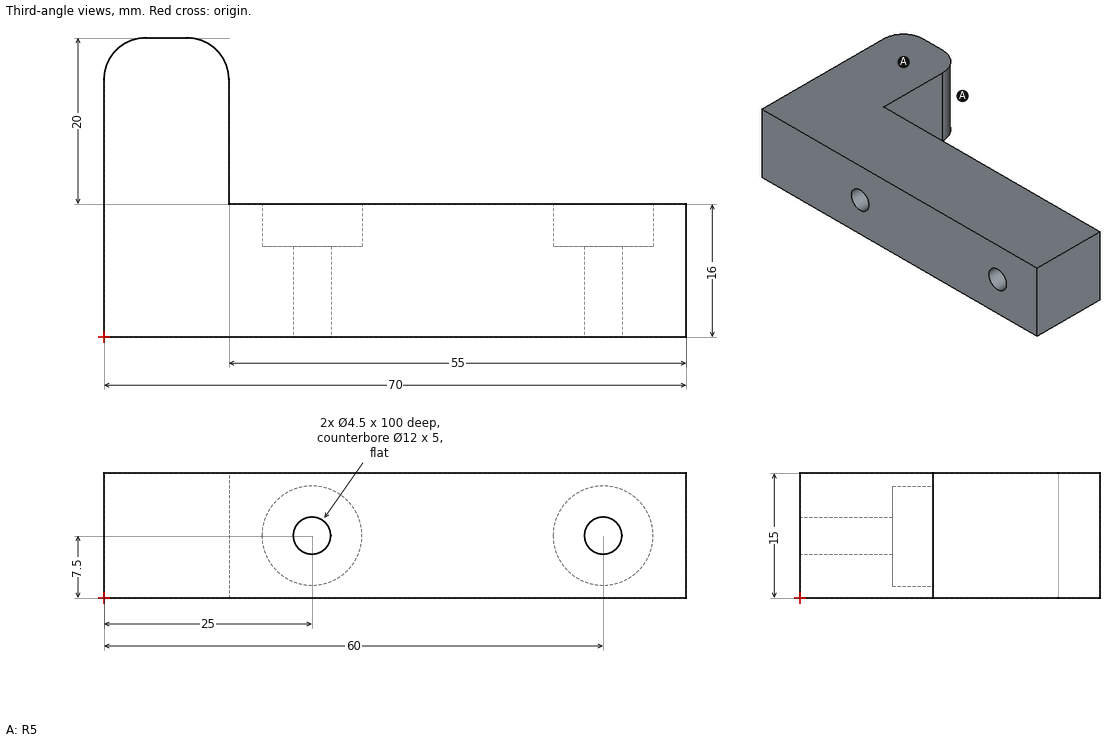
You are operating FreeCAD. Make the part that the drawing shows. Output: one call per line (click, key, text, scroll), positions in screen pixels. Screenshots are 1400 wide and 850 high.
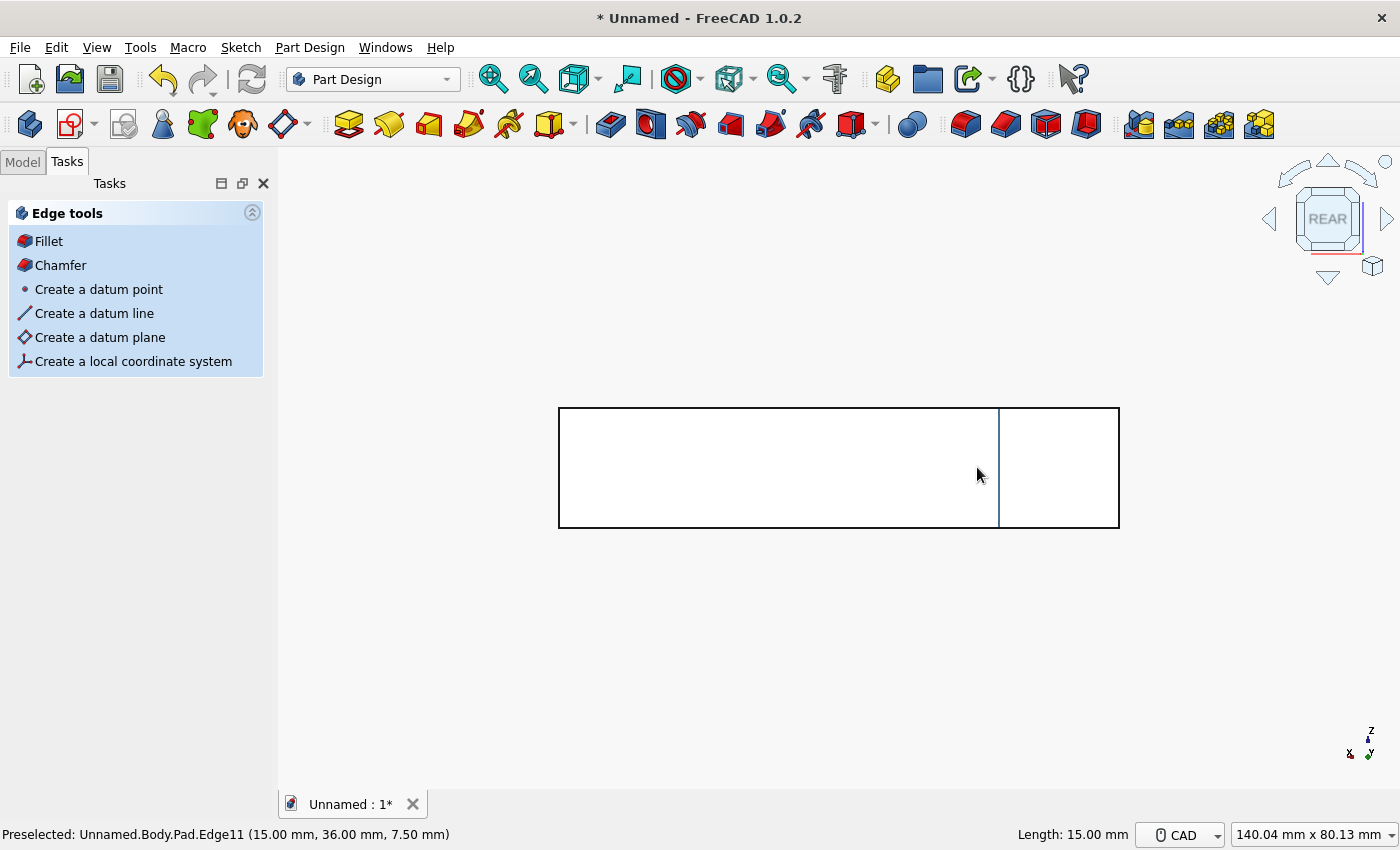
click(1119, 467, ctrl)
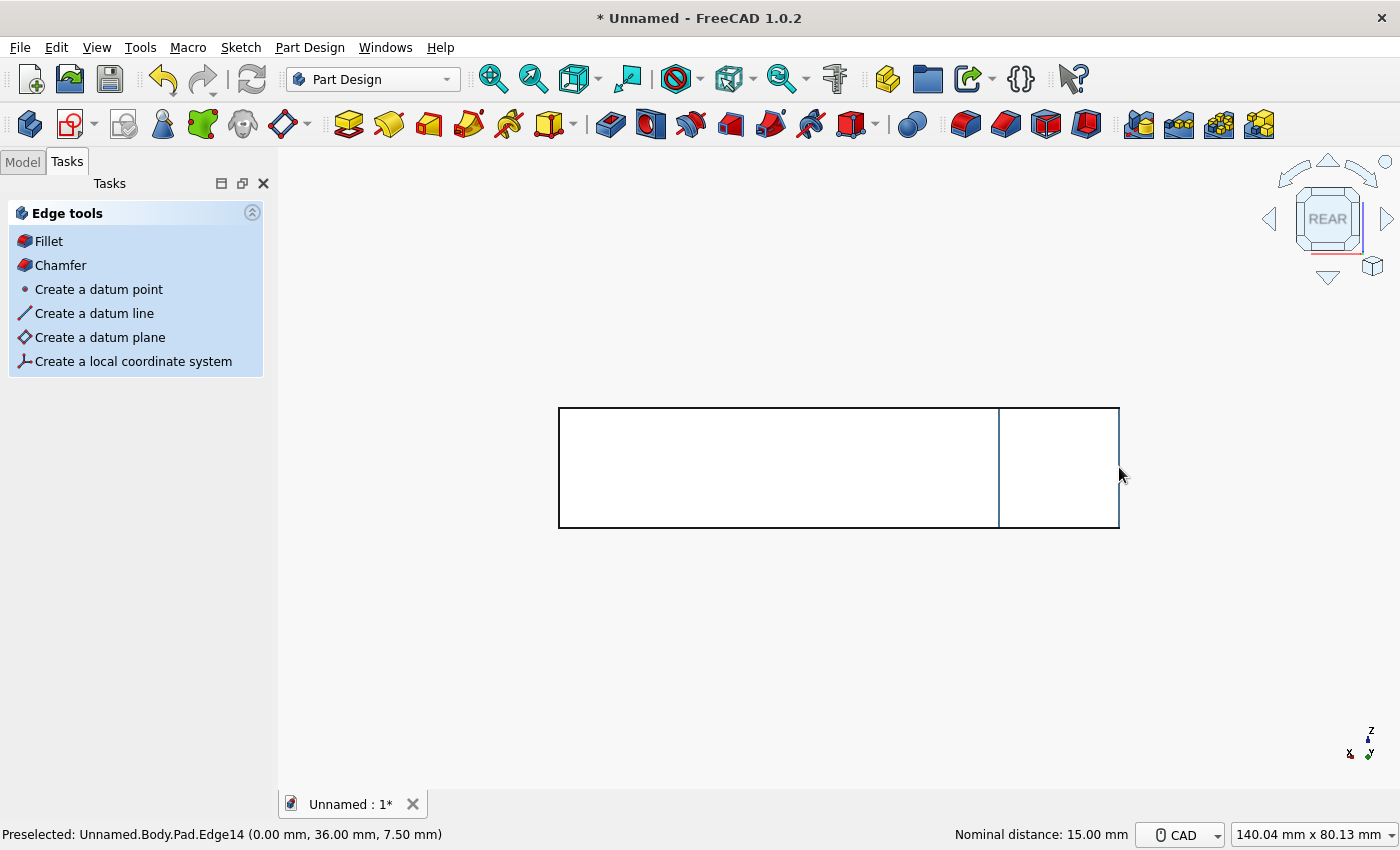
click(966, 124)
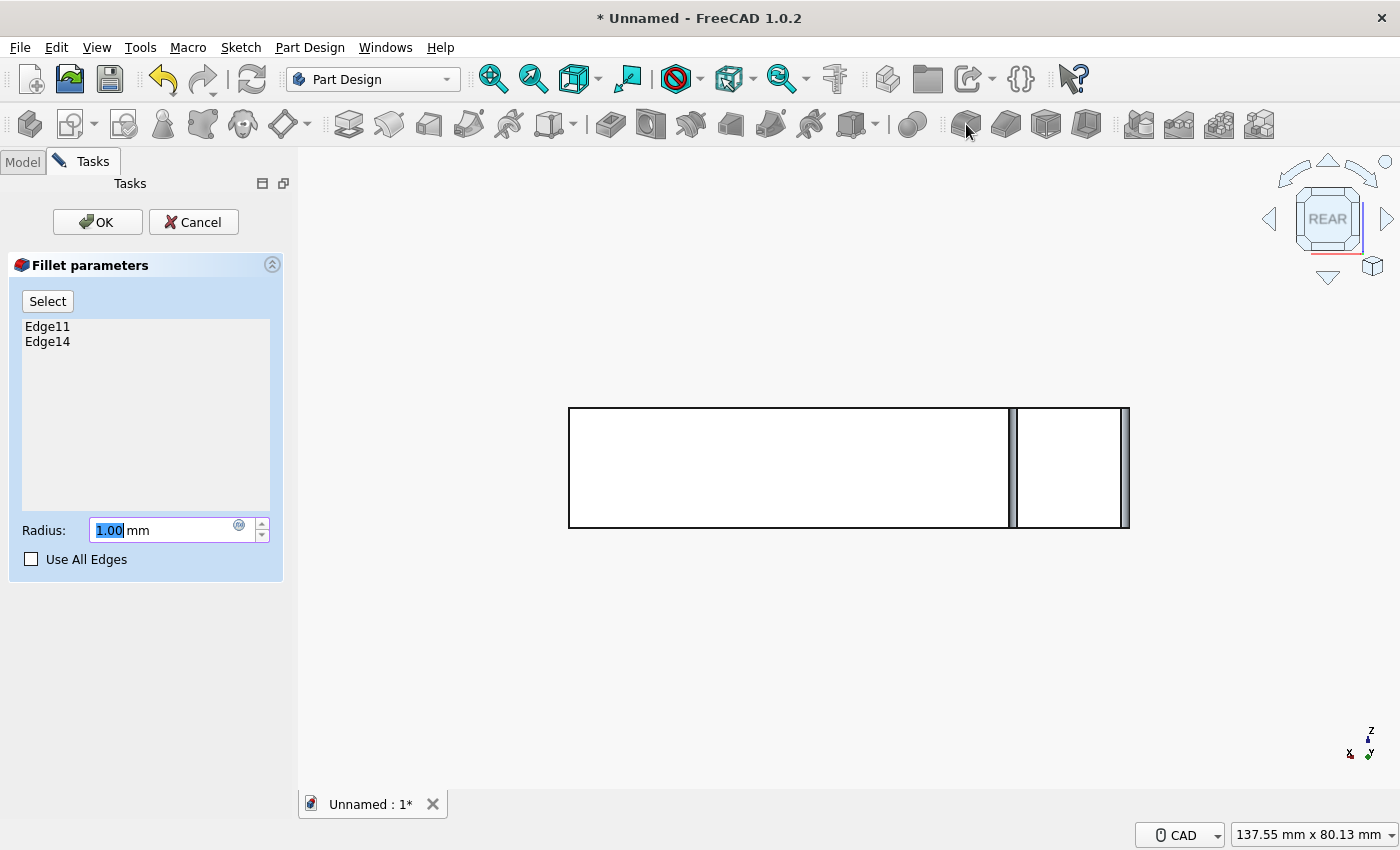
text(5)
key(Tab)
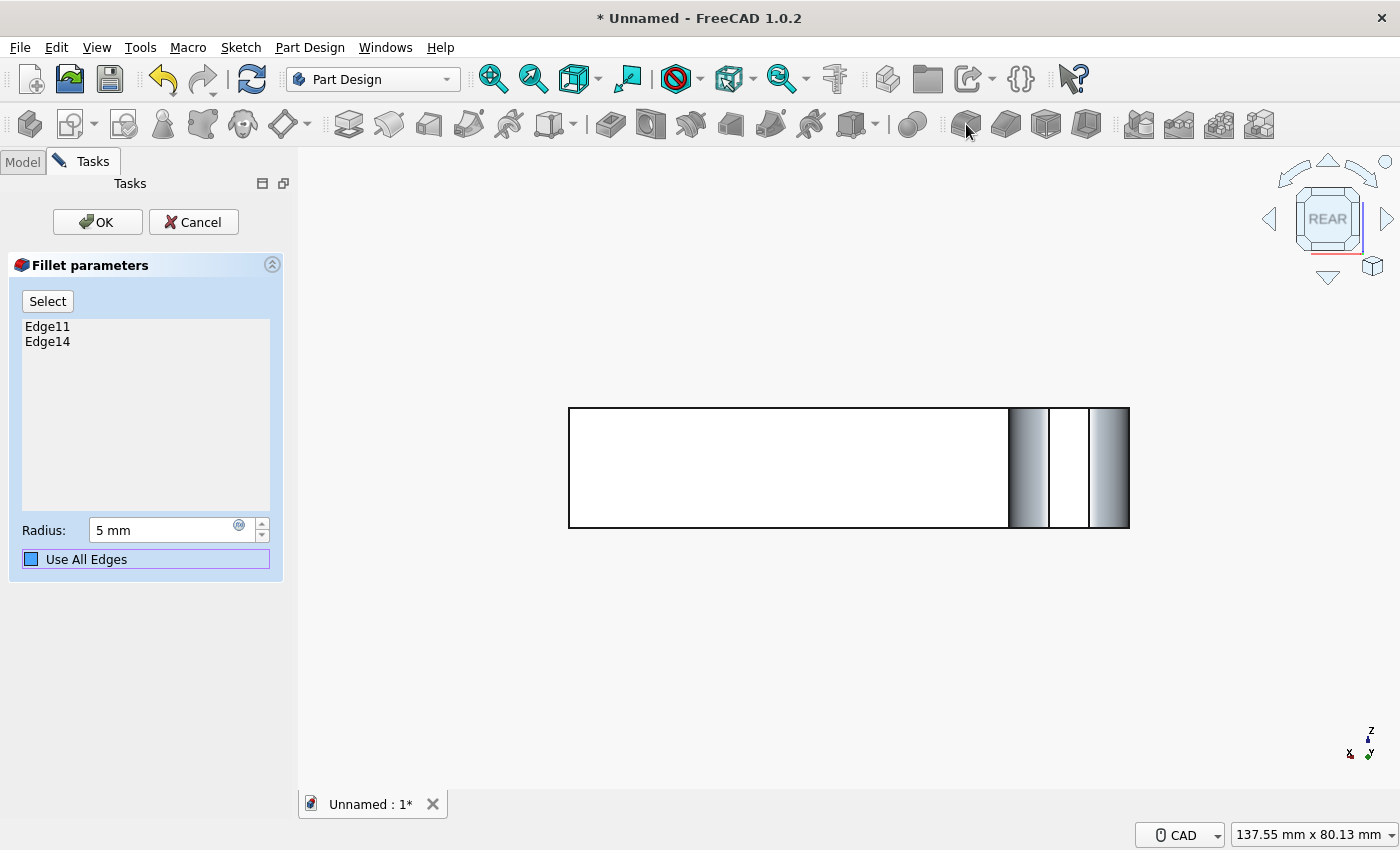
click(98, 222)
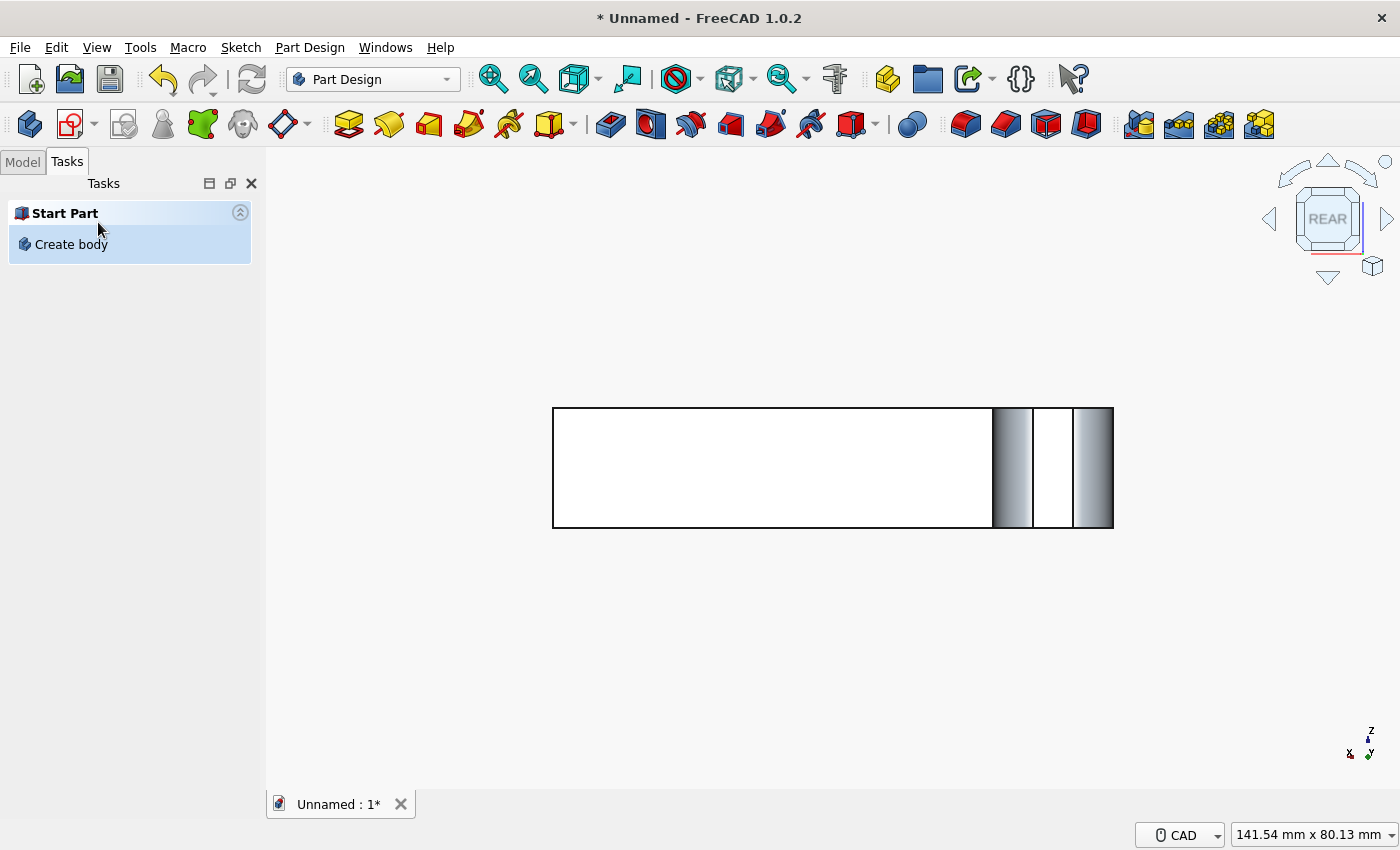
click(647, 467)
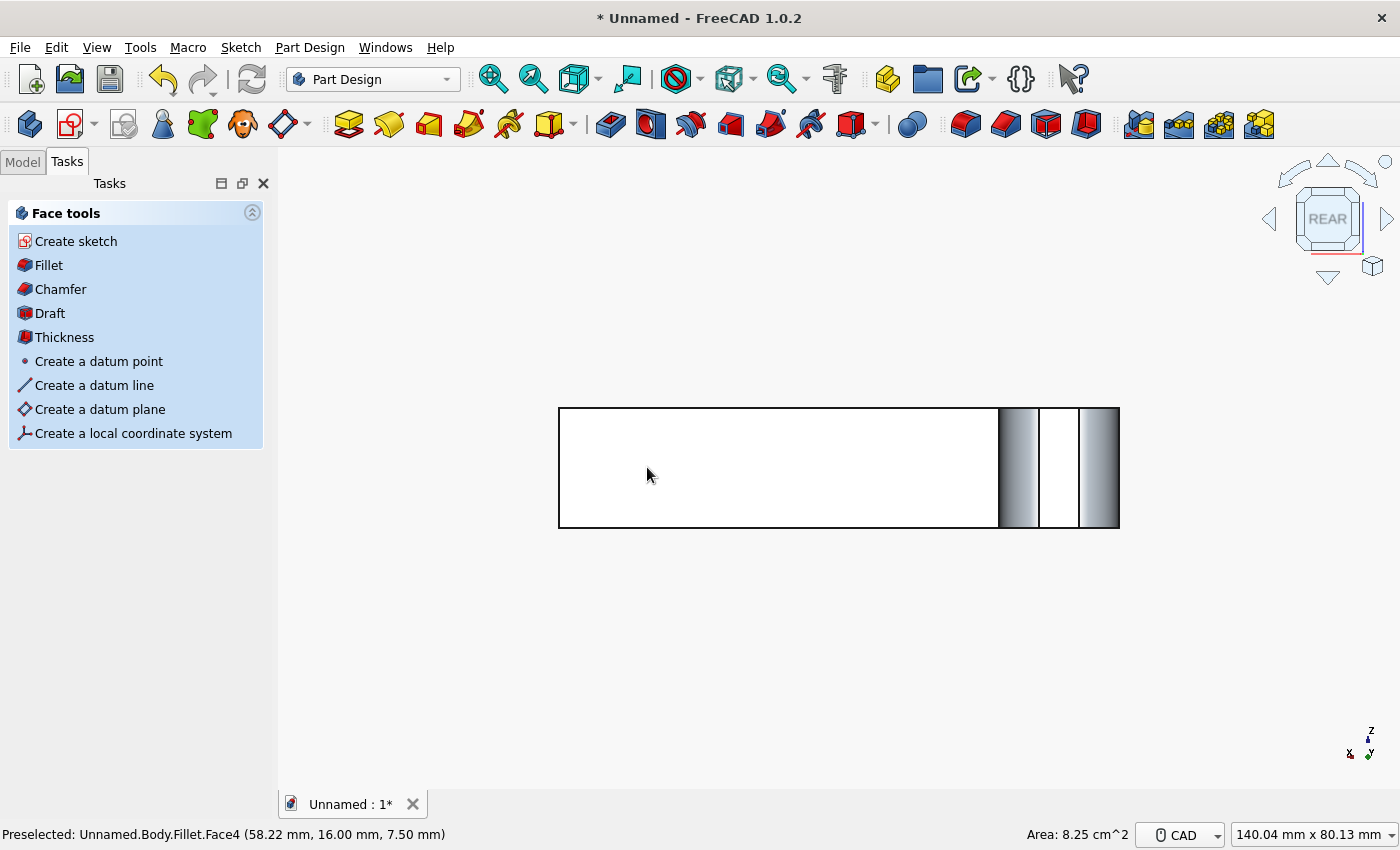
click(70, 124)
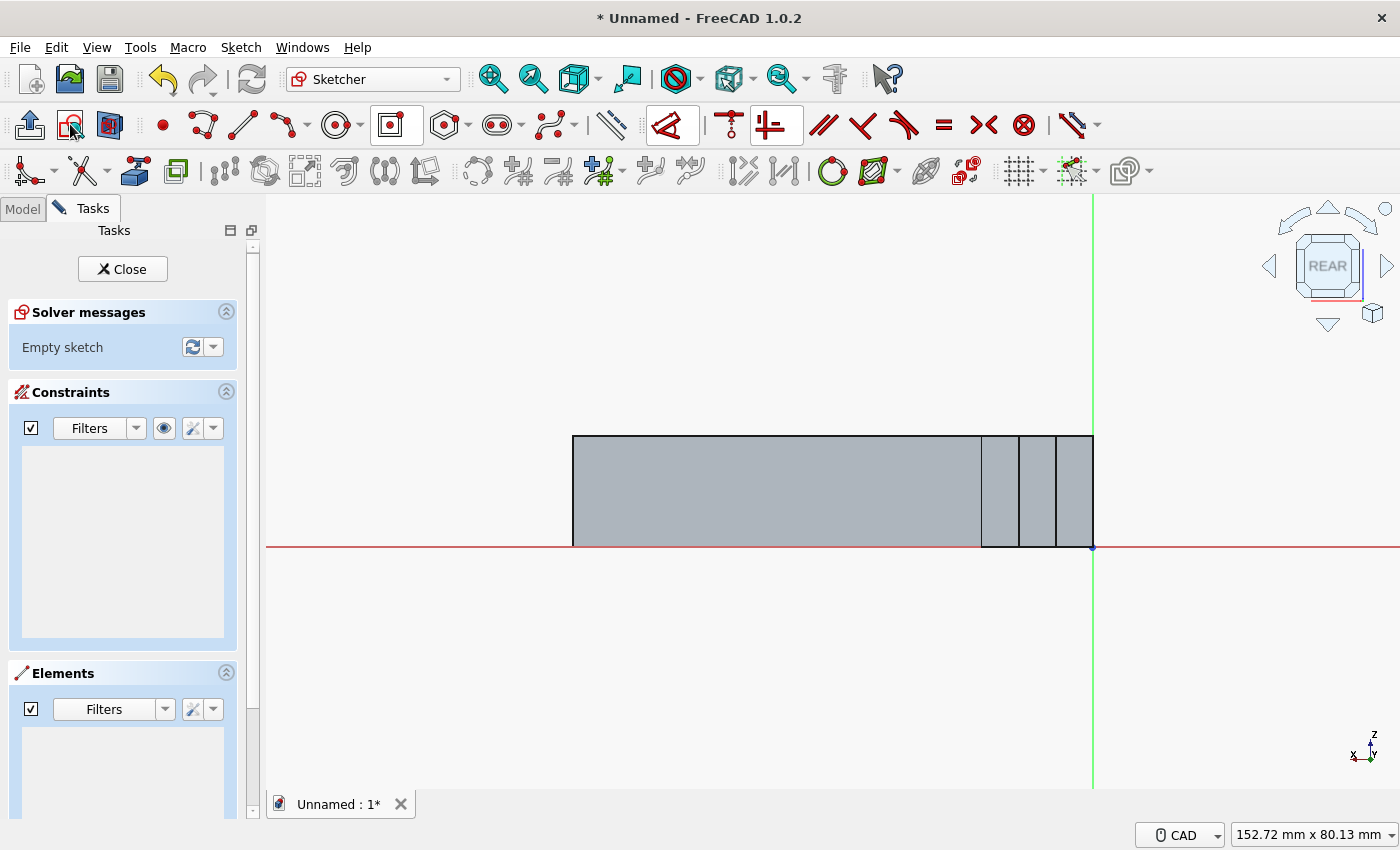
click(110, 126)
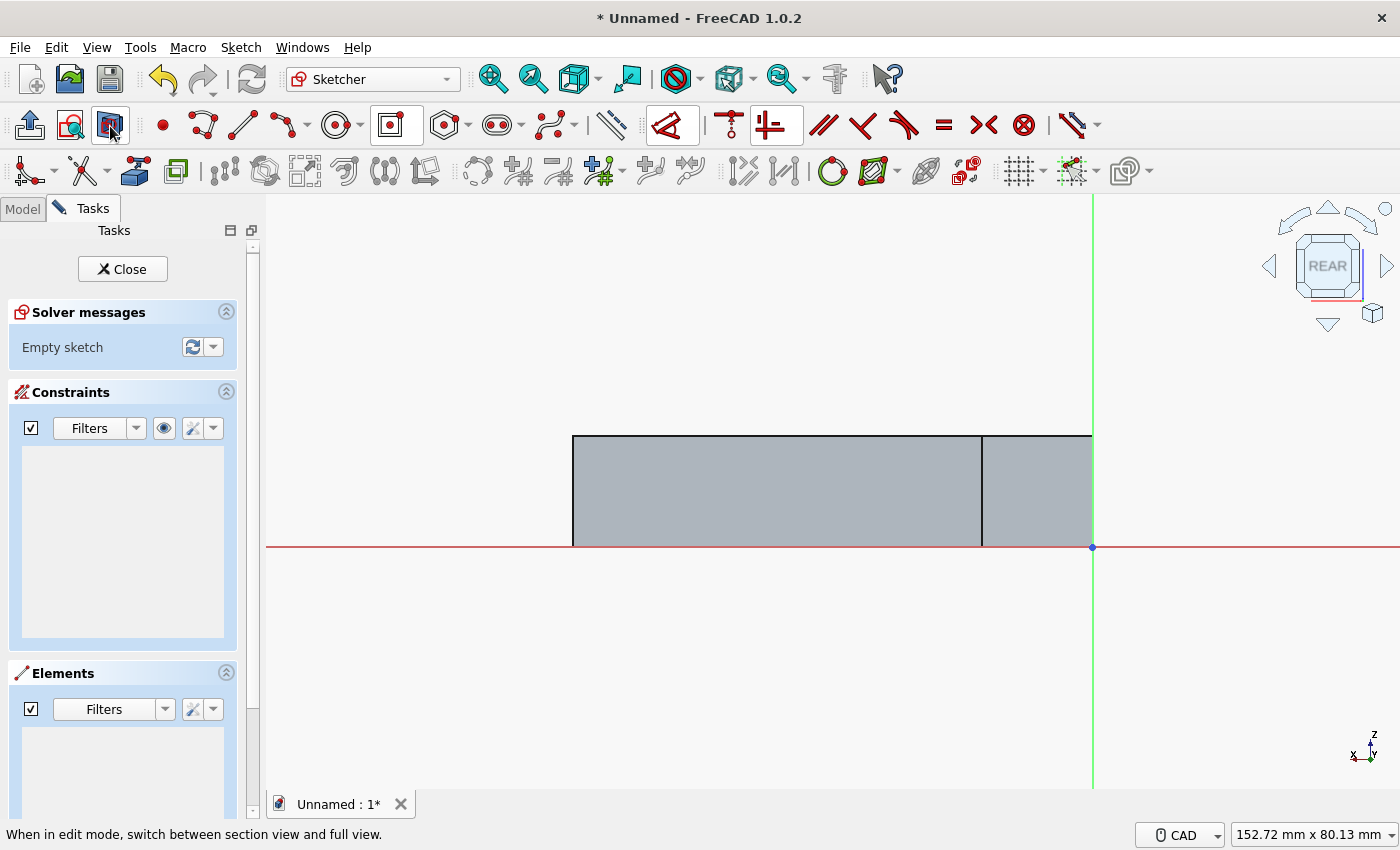
scroll(1060, 551, up, 2)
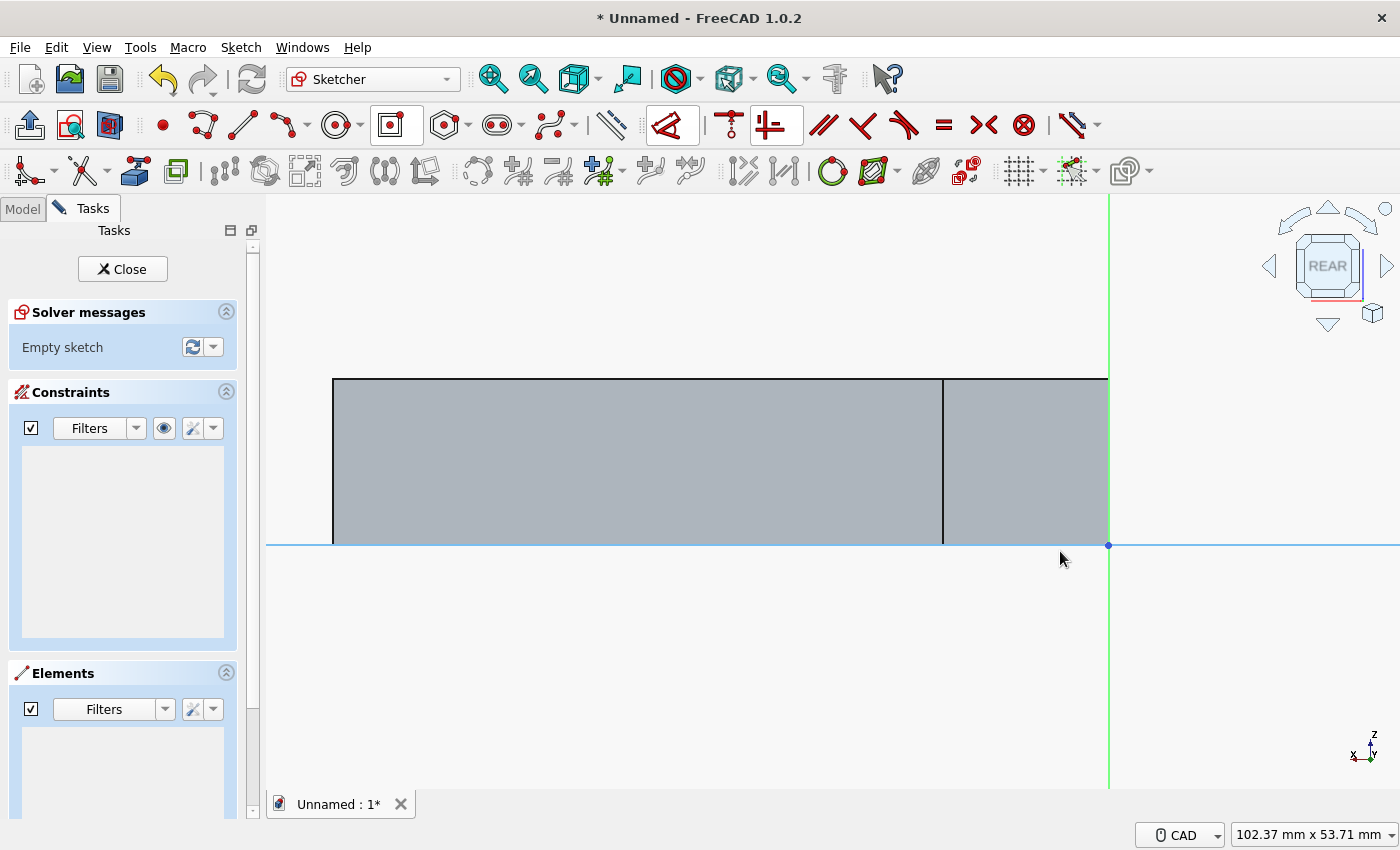
click(336, 126)